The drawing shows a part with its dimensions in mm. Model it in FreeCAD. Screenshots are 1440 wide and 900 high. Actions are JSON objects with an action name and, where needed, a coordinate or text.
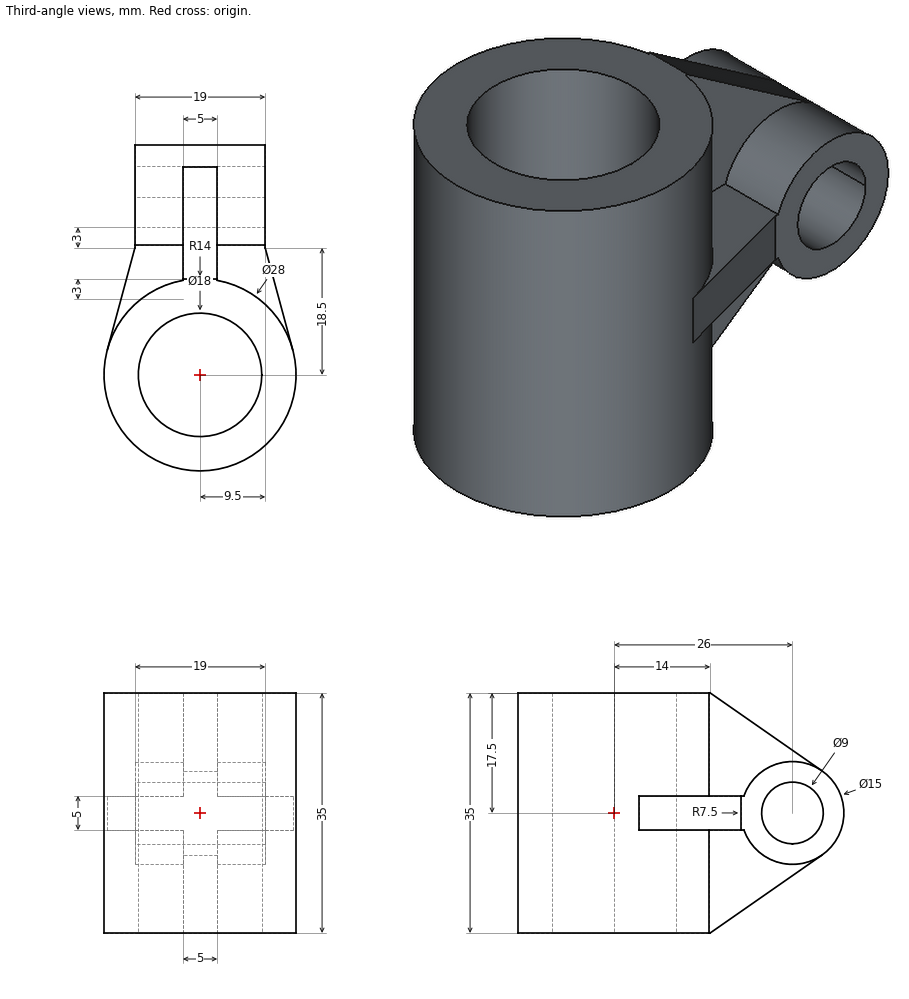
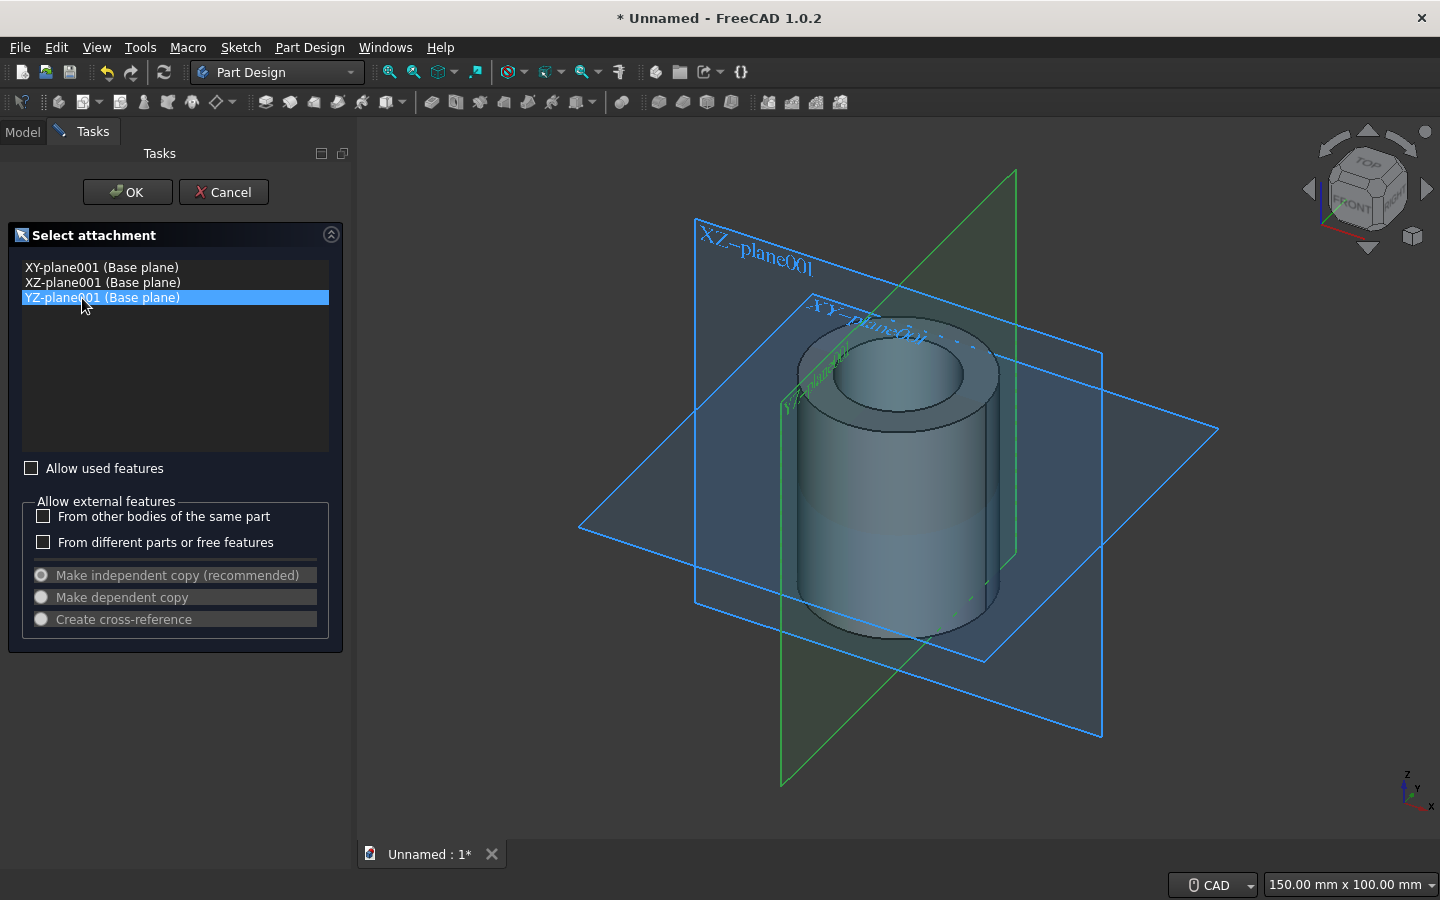
{"action": "left_click", "coordinate": [128, 192]}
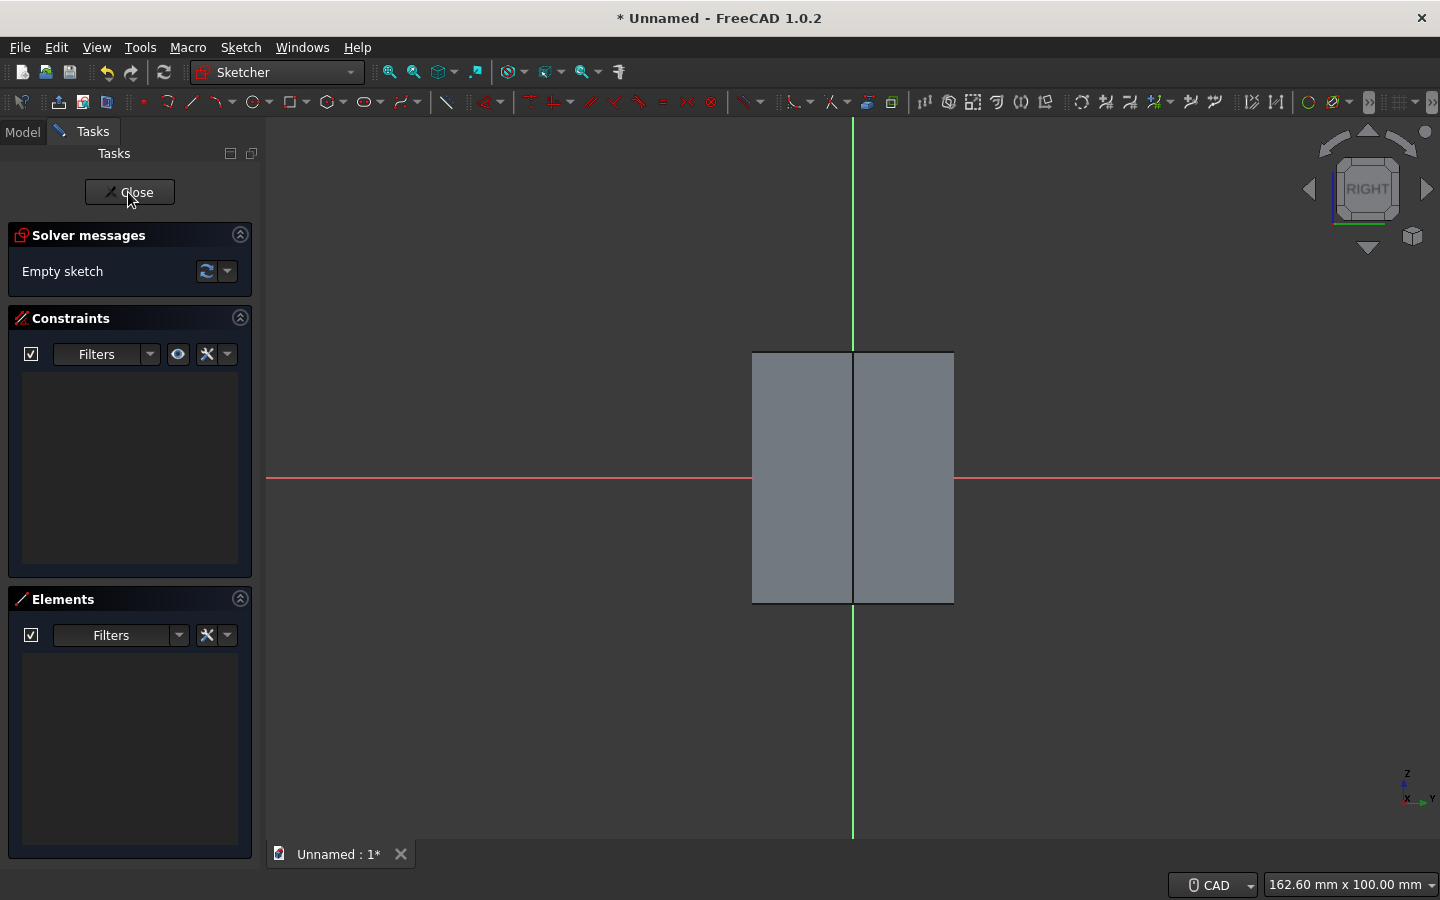
{"action": "scroll", "coordinate": [1084, 478], "scroll_direction": "up", "scroll_amount": 5}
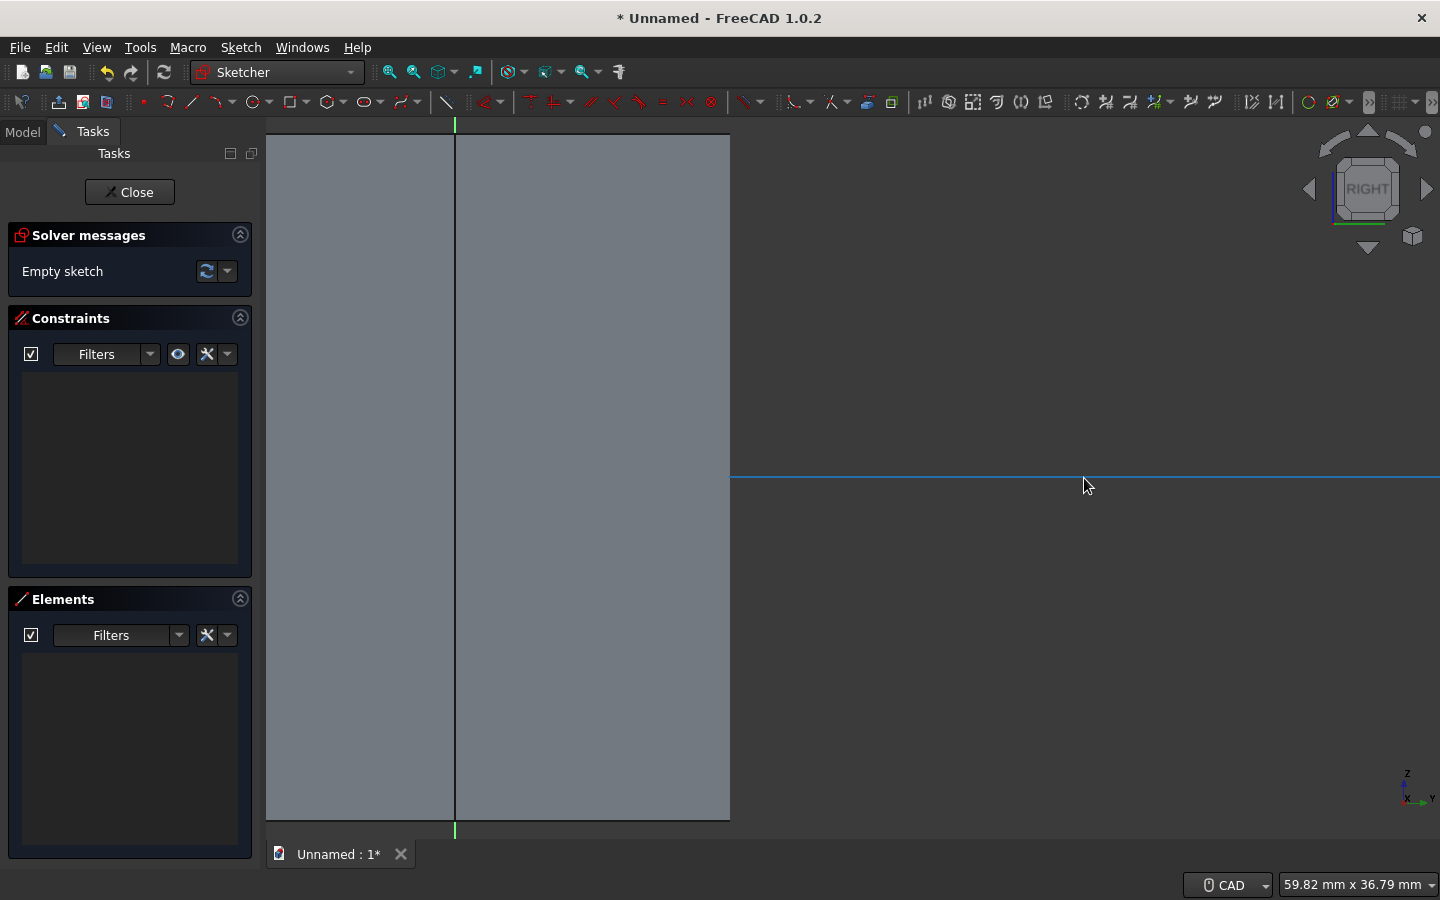
{"action": "left_click", "coordinate": [254, 102]}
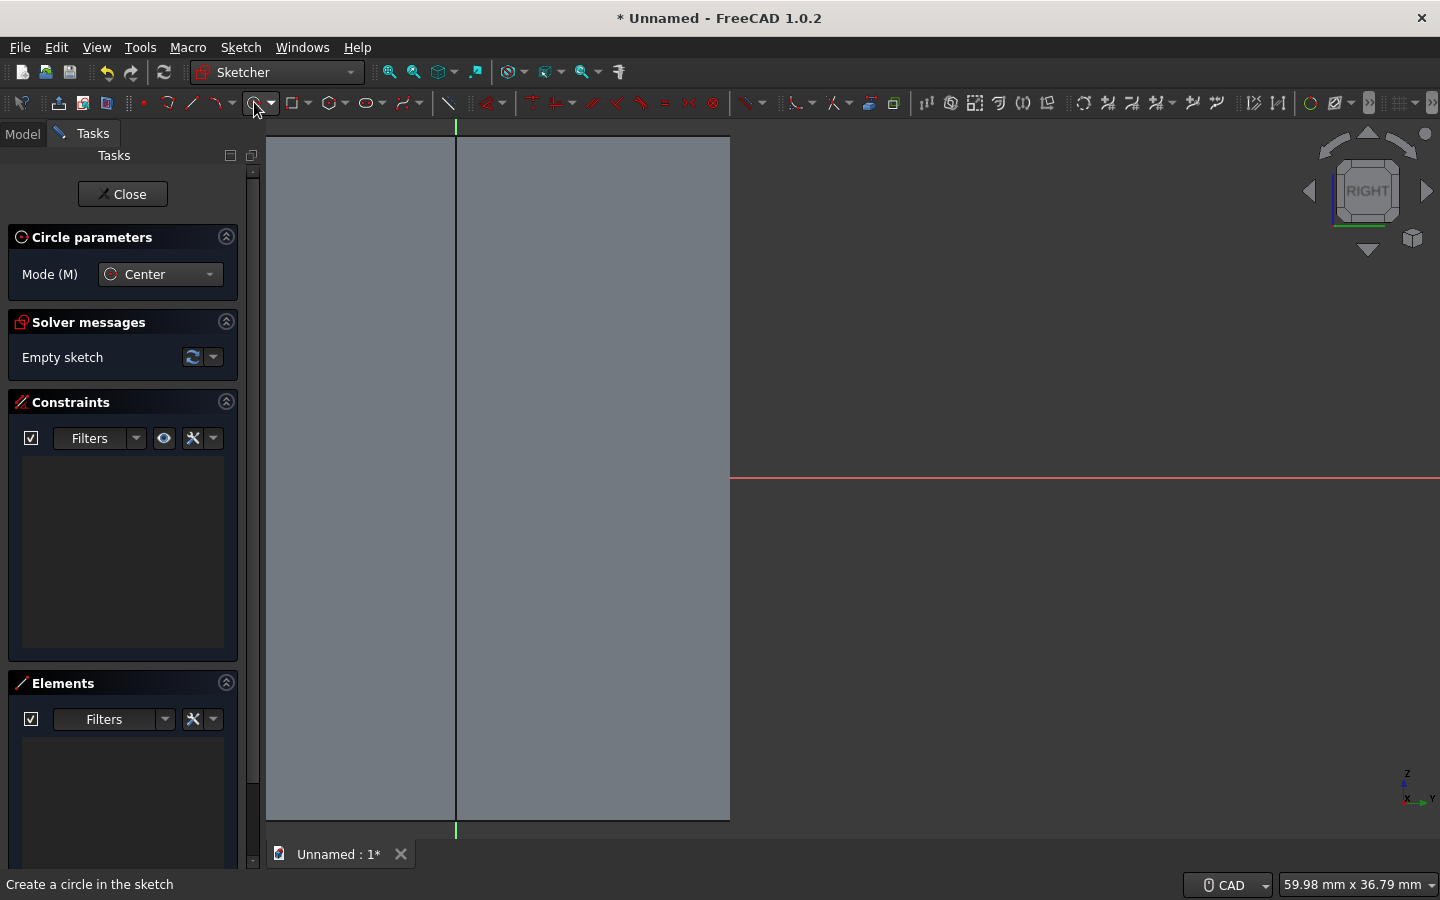
{"action": "left_click", "coordinate": [965, 478]}
{"action": "left_click", "coordinate": [1069, 374]}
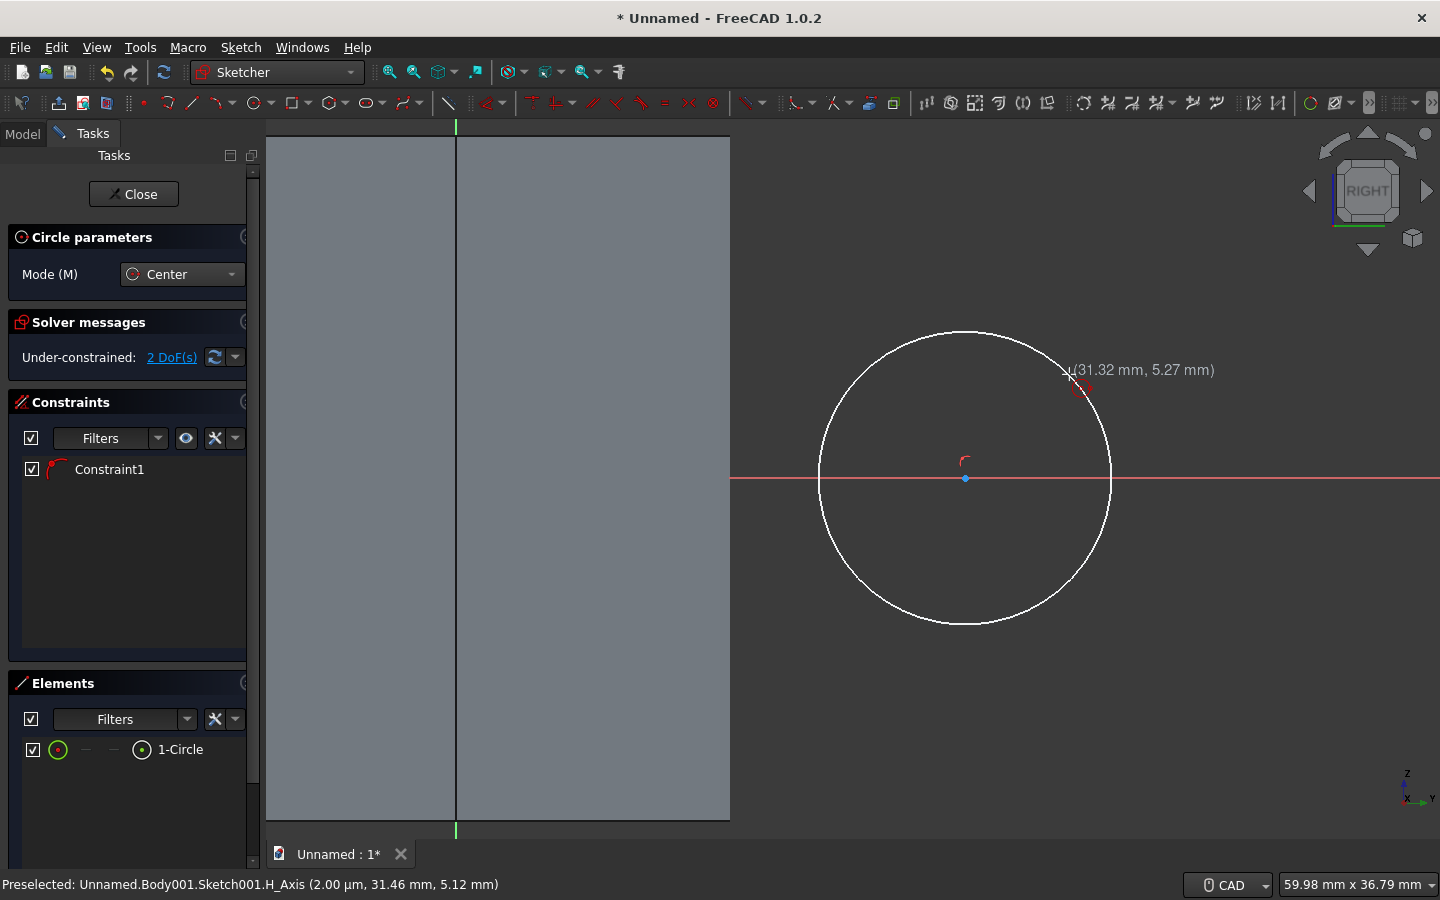
{"action": "left_click", "coordinate": [965, 478]}
{"action": "left_click", "coordinate": [1027, 416]}
{"action": "key", "text": "Escape"}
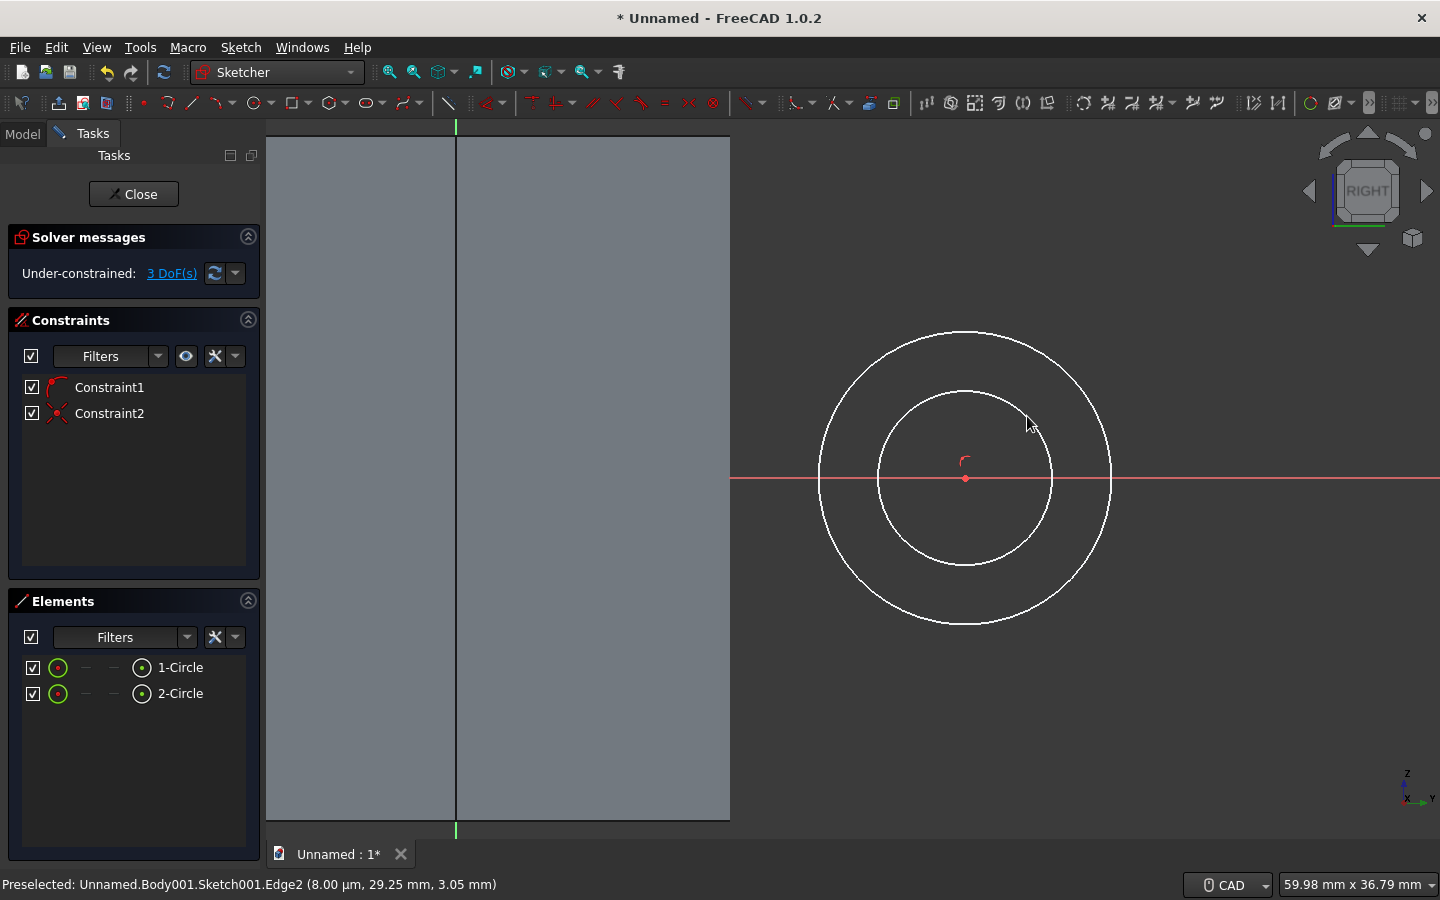
{"action": "key", "text": "d"}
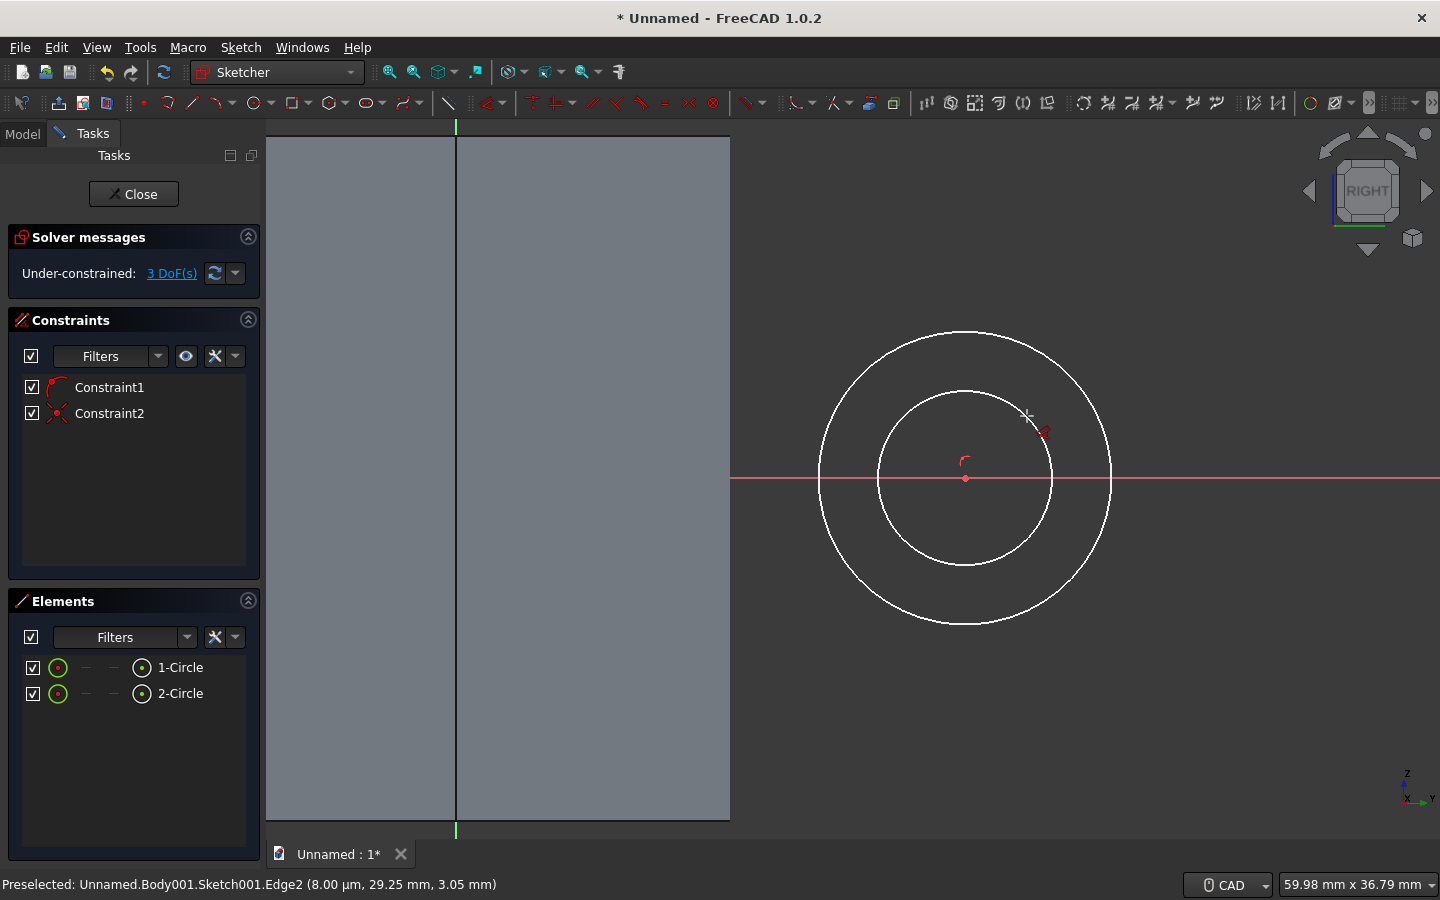
{"action": "left_click", "coordinate": [1068, 374]}
{"action": "left_click", "coordinate": [1091, 351]}